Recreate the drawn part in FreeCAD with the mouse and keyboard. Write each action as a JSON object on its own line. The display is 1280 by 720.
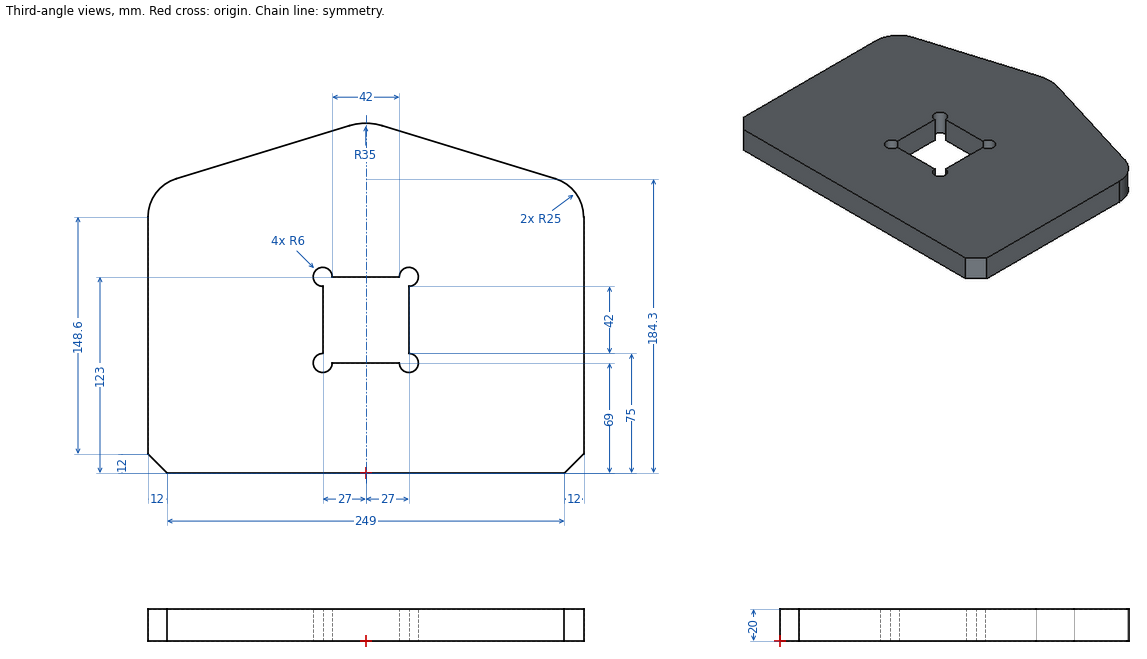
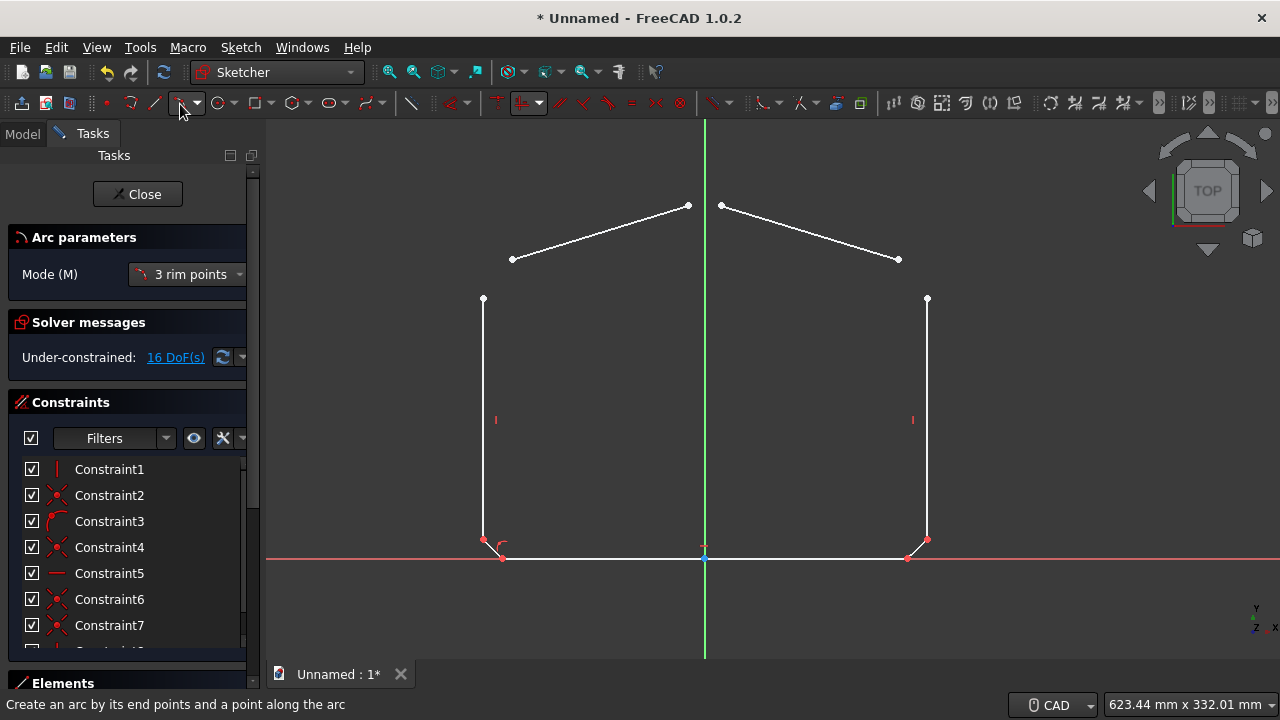
{"action": "left_click", "coordinate": [721, 206]}
{"action": "left_click", "coordinate": [688, 206]}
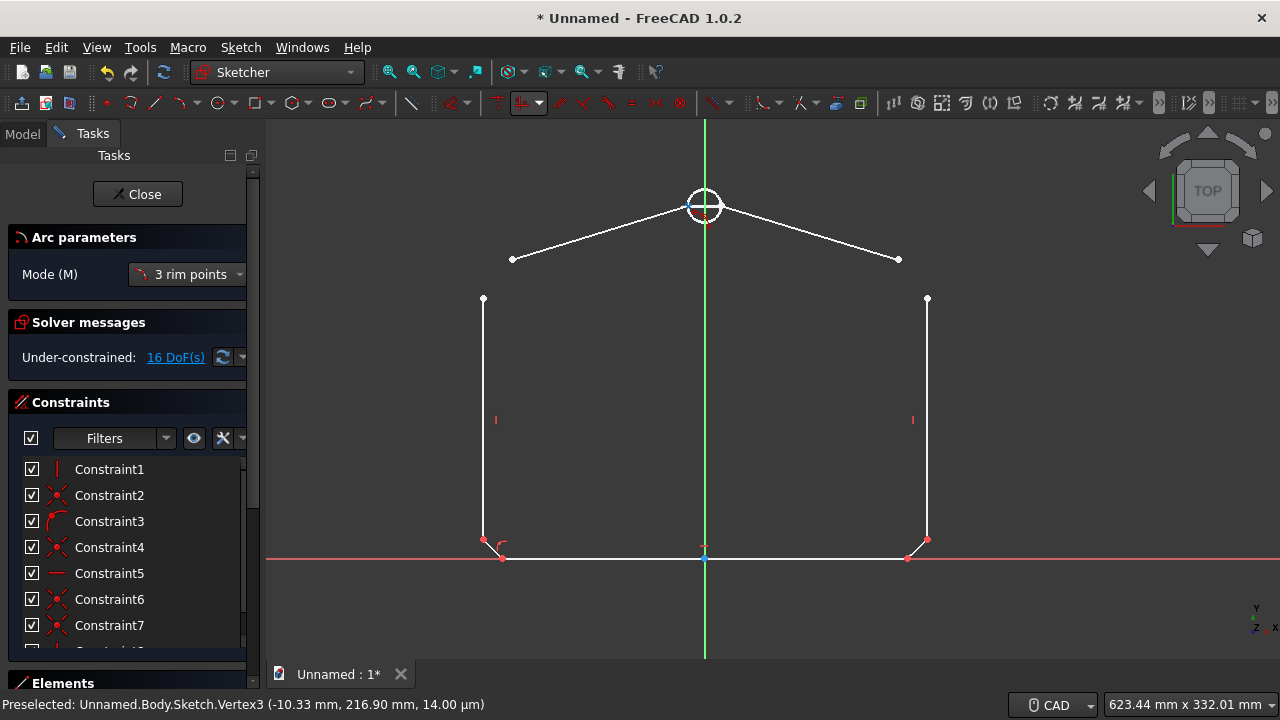
{"action": "scroll", "coordinate": [708, 202], "scroll_direction": "up", "scroll_amount": 10}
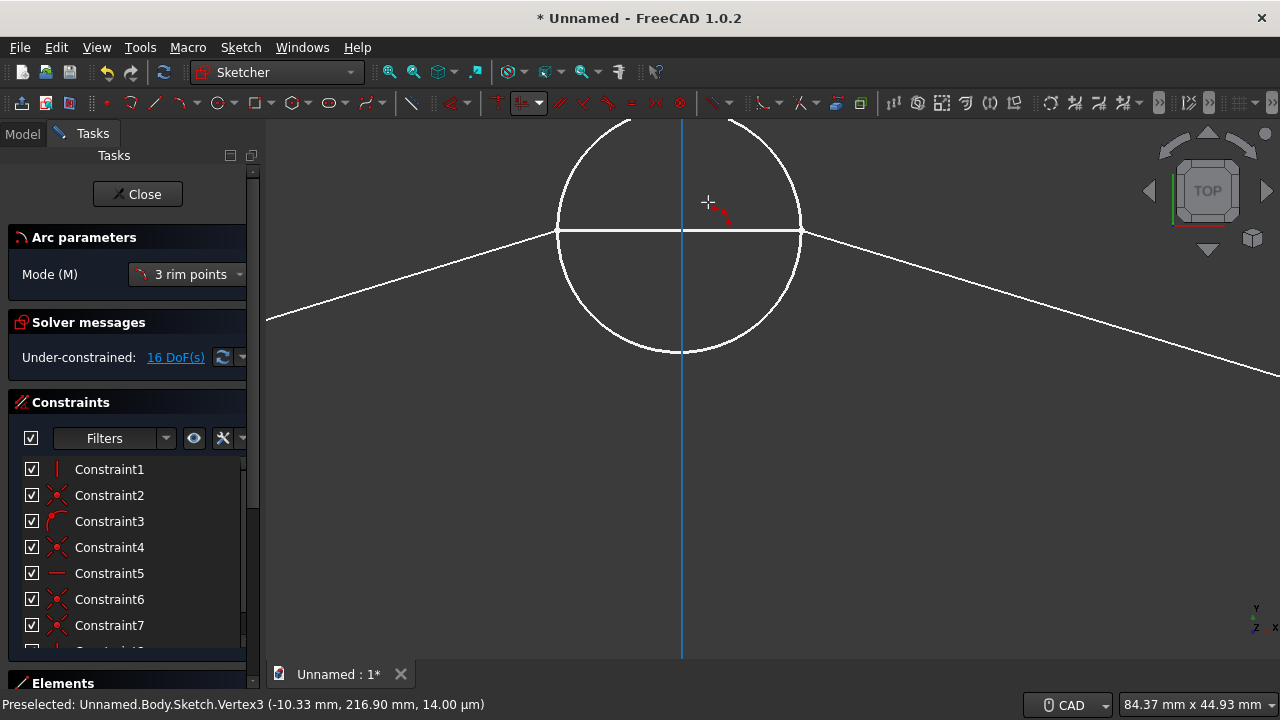
{"action": "left_click", "coordinate": [707, 202]}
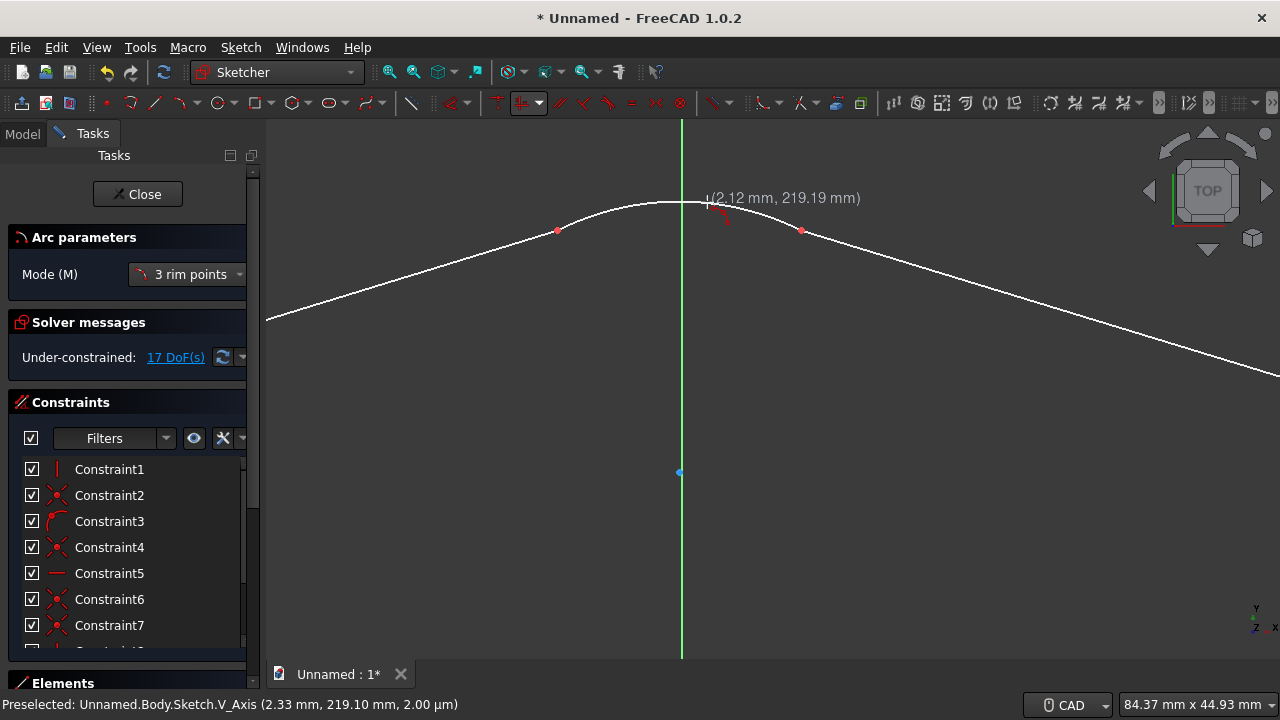
{"action": "scroll", "coordinate": [708, 212], "scroll_direction": "down", "scroll_amount": 10}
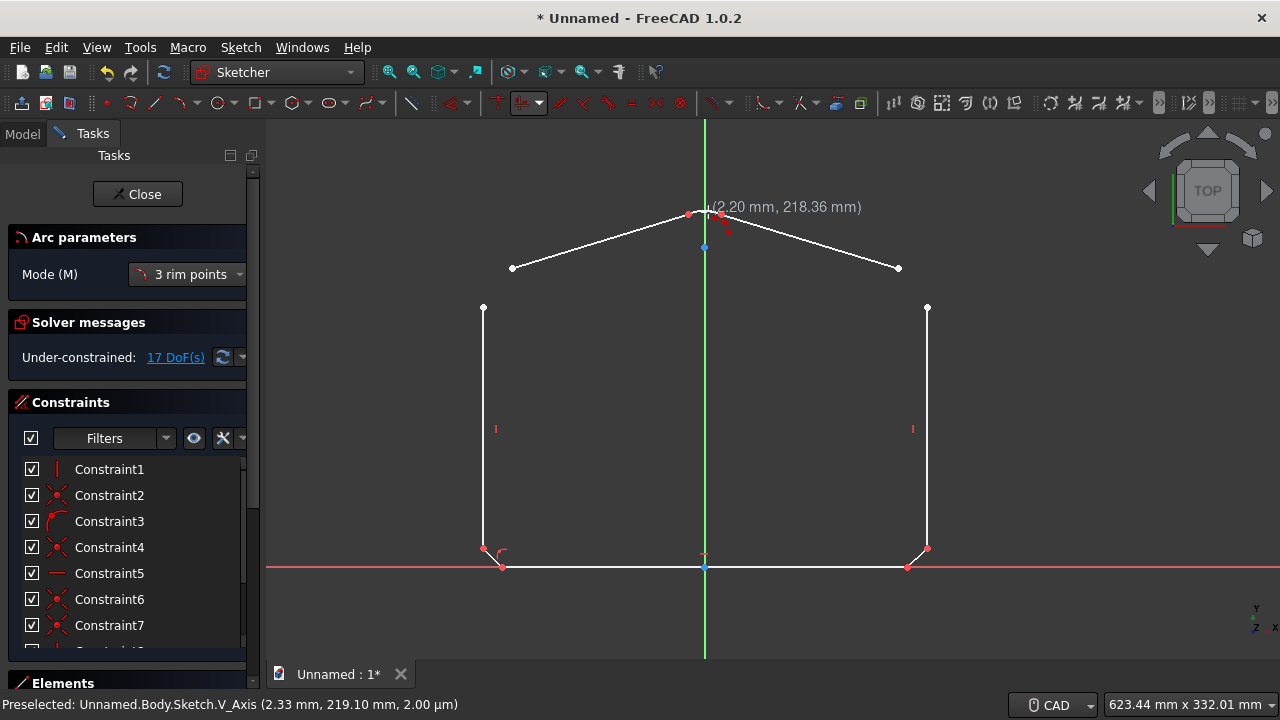
{"action": "left_click", "coordinate": [512, 269]}
{"action": "left_click", "coordinate": [483, 308]}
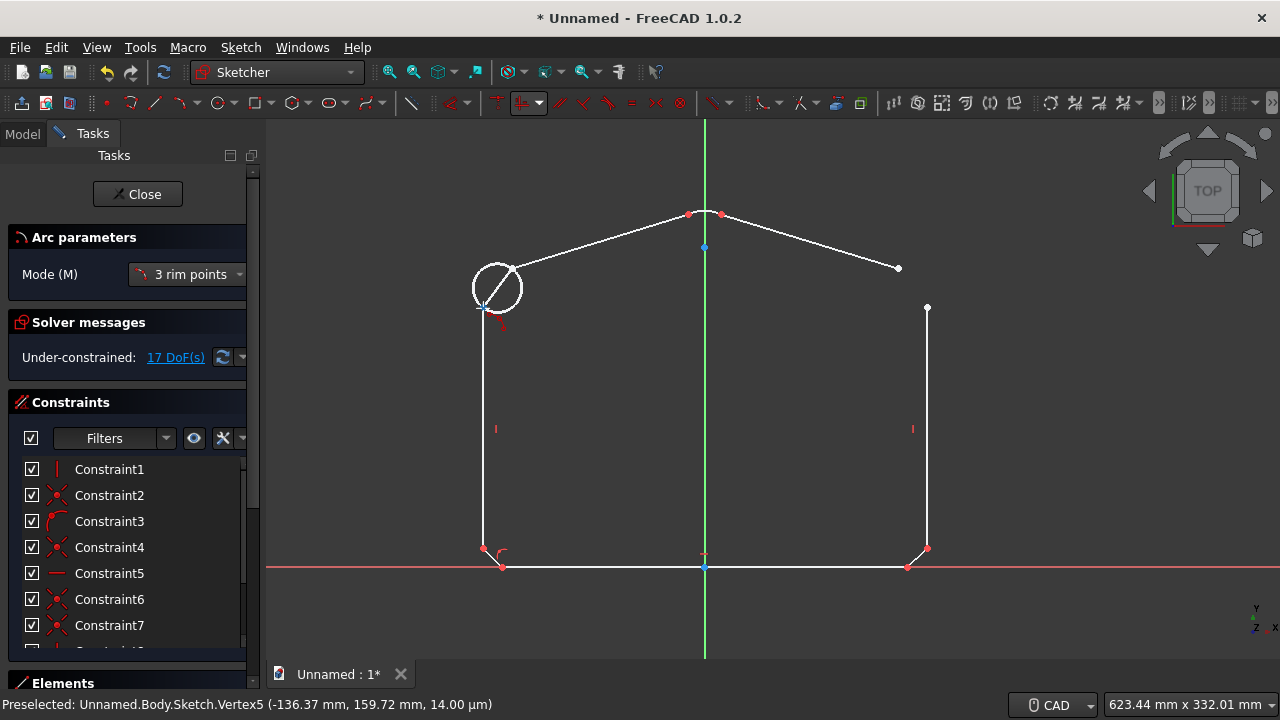
{"action": "scroll", "coordinate": [491, 282], "scroll_direction": "up", "scroll_amount": 4}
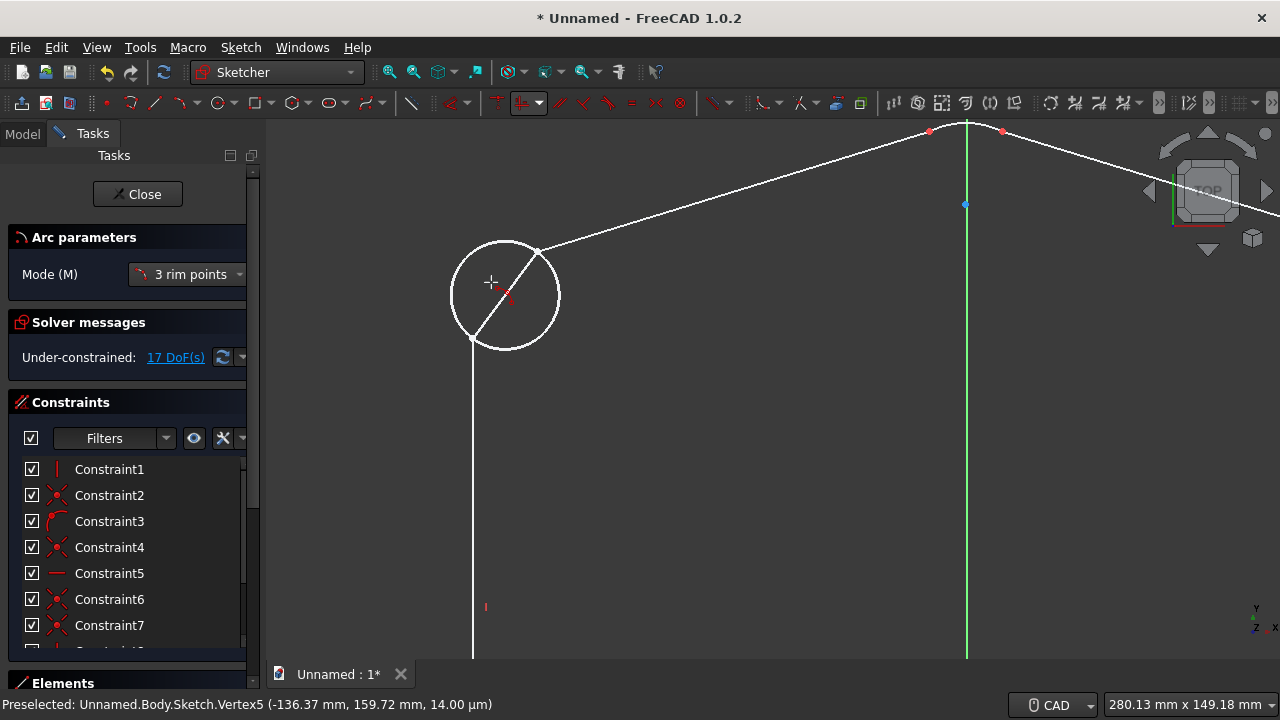
{"action": "left_click", "coordinate": [490, 282]}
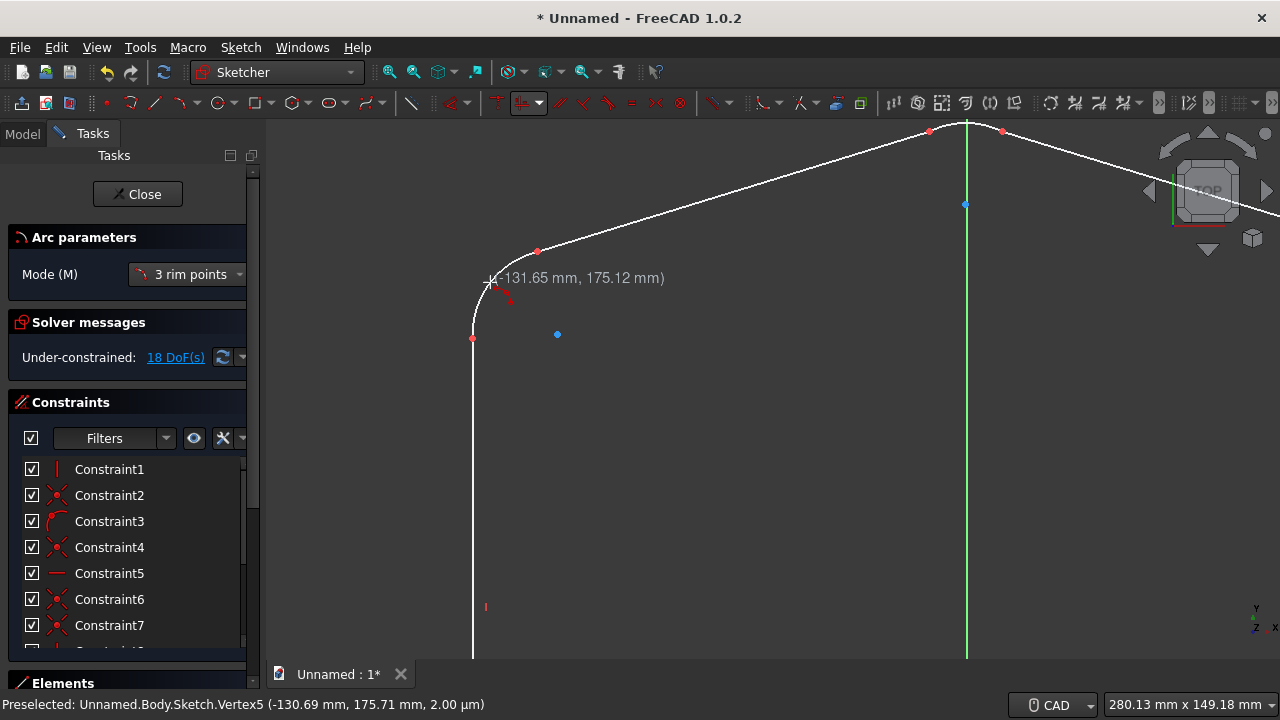
{"action": "scroll", "coordinate": [491, 282], "scroll_direction": "down", "scroll_amount": 4}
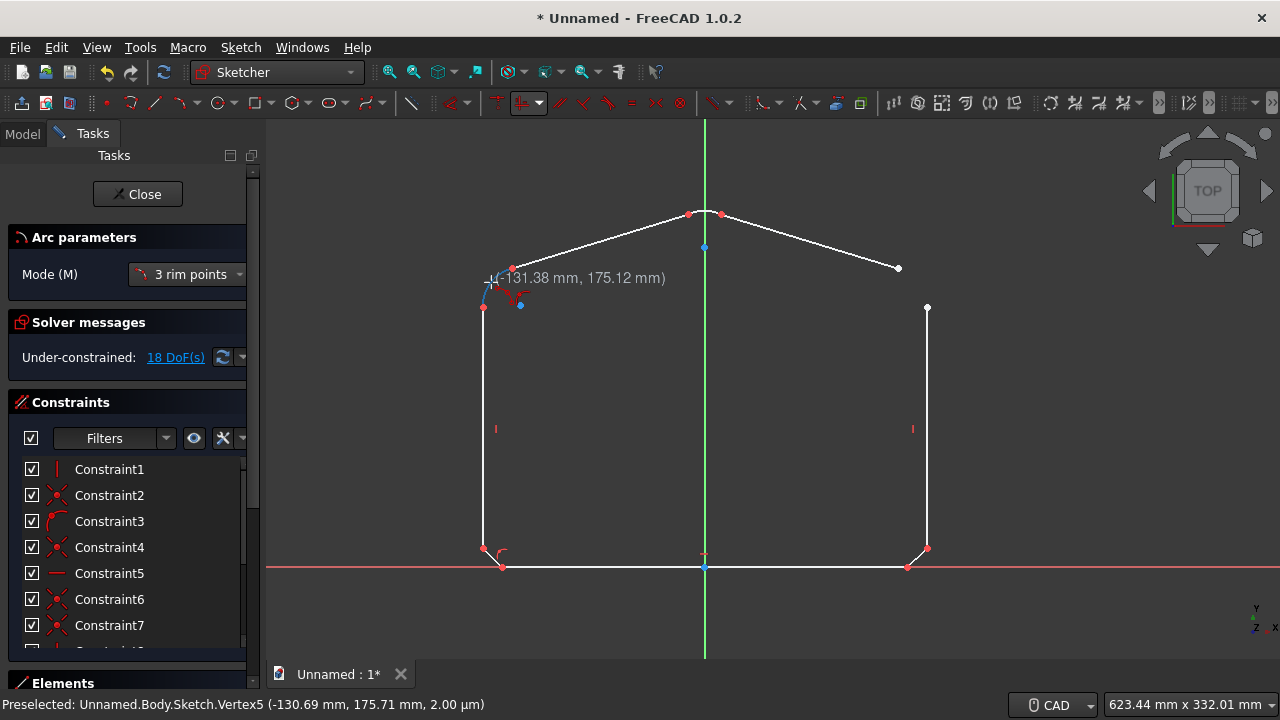
{"action": "left_click", "coordinate": [927, 308]}
{"action": "left_click", "coordinate": [898, 269]}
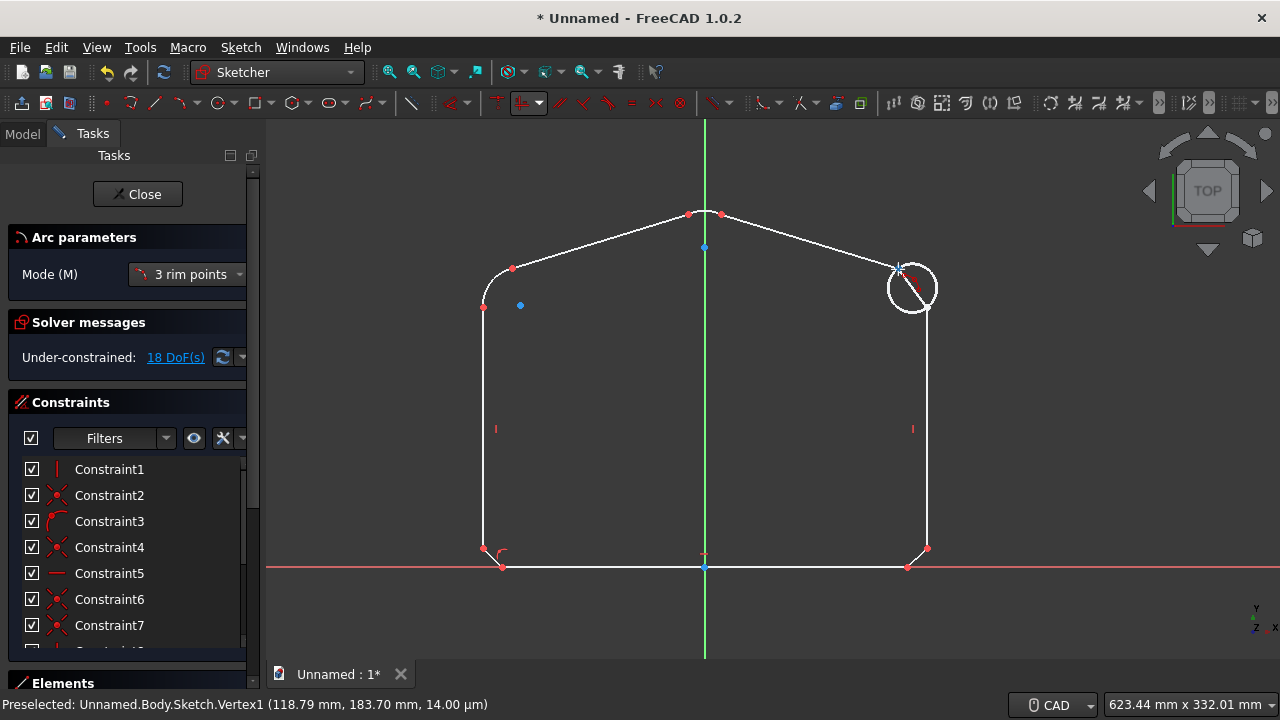
{"action": "scroll", "coordinate": [919, 282], "scroll_direction": "up", "scroll_amount": 4}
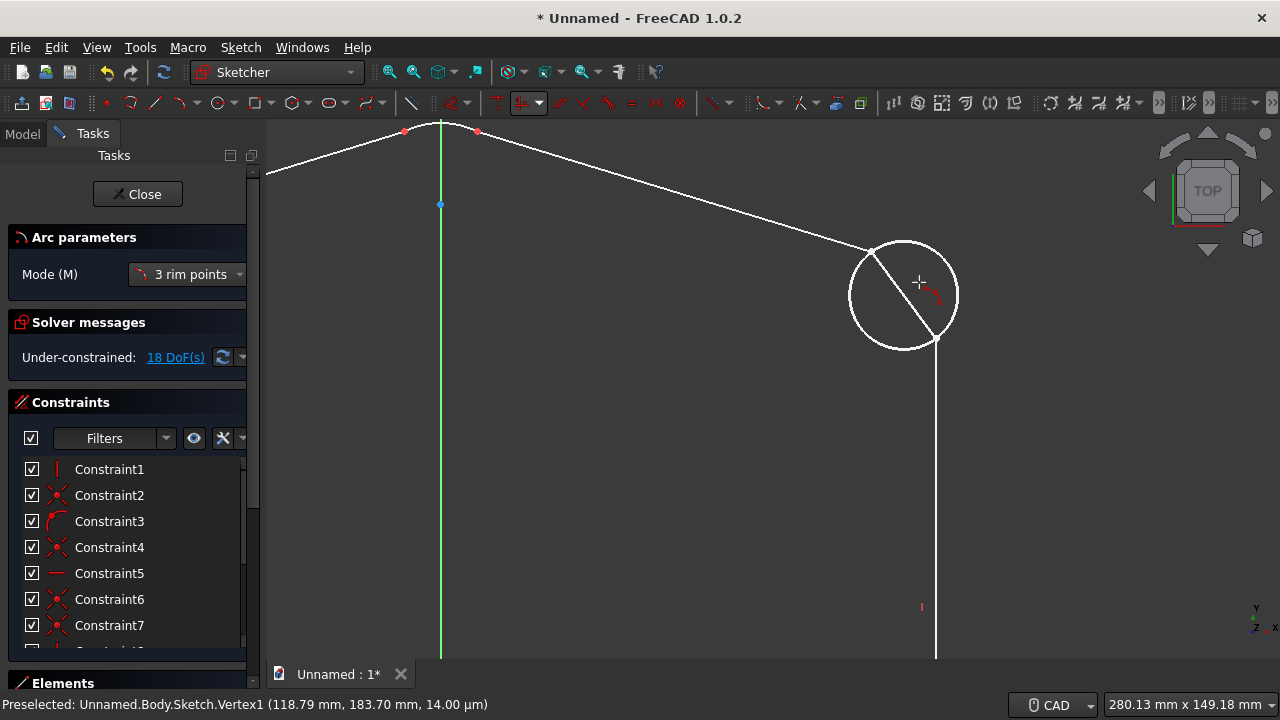
{"action": "left_click", "coordinate": [918, 282]}